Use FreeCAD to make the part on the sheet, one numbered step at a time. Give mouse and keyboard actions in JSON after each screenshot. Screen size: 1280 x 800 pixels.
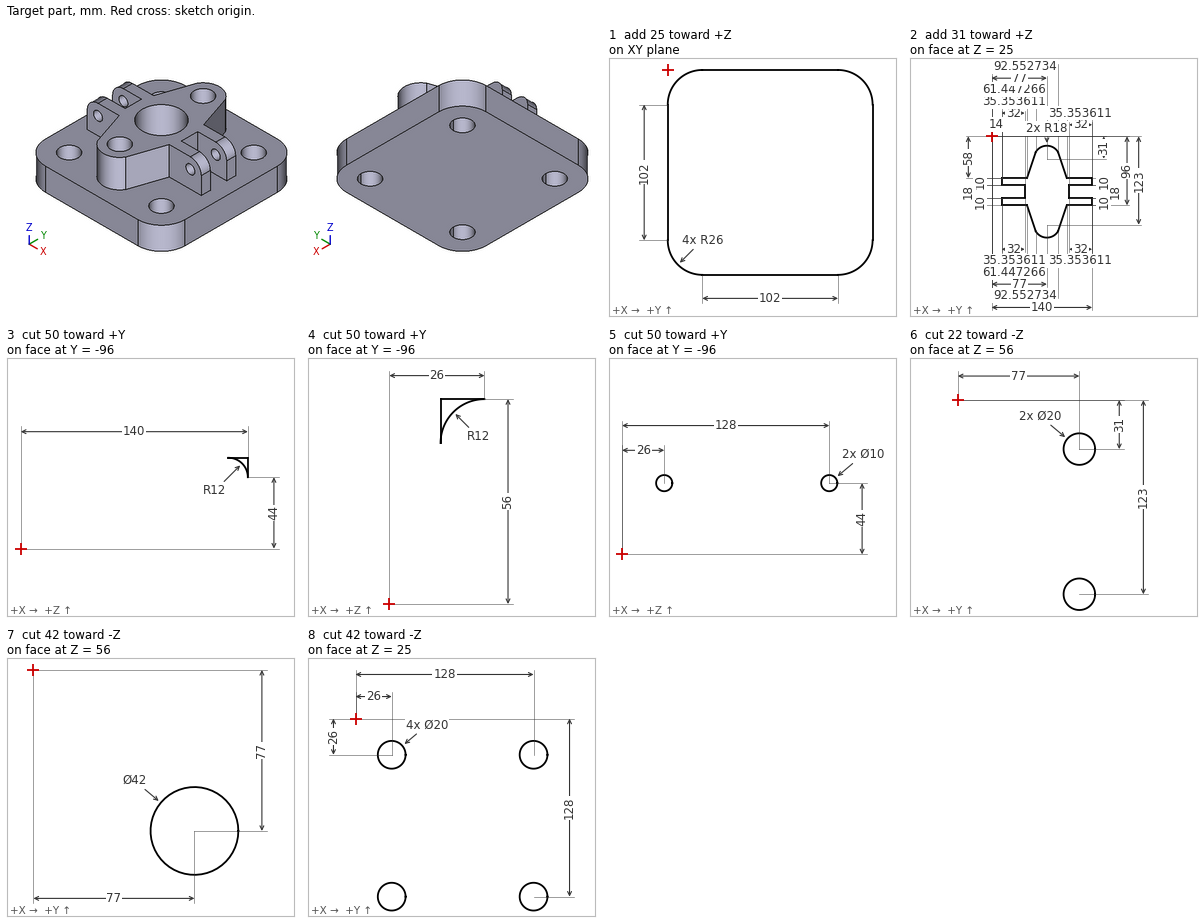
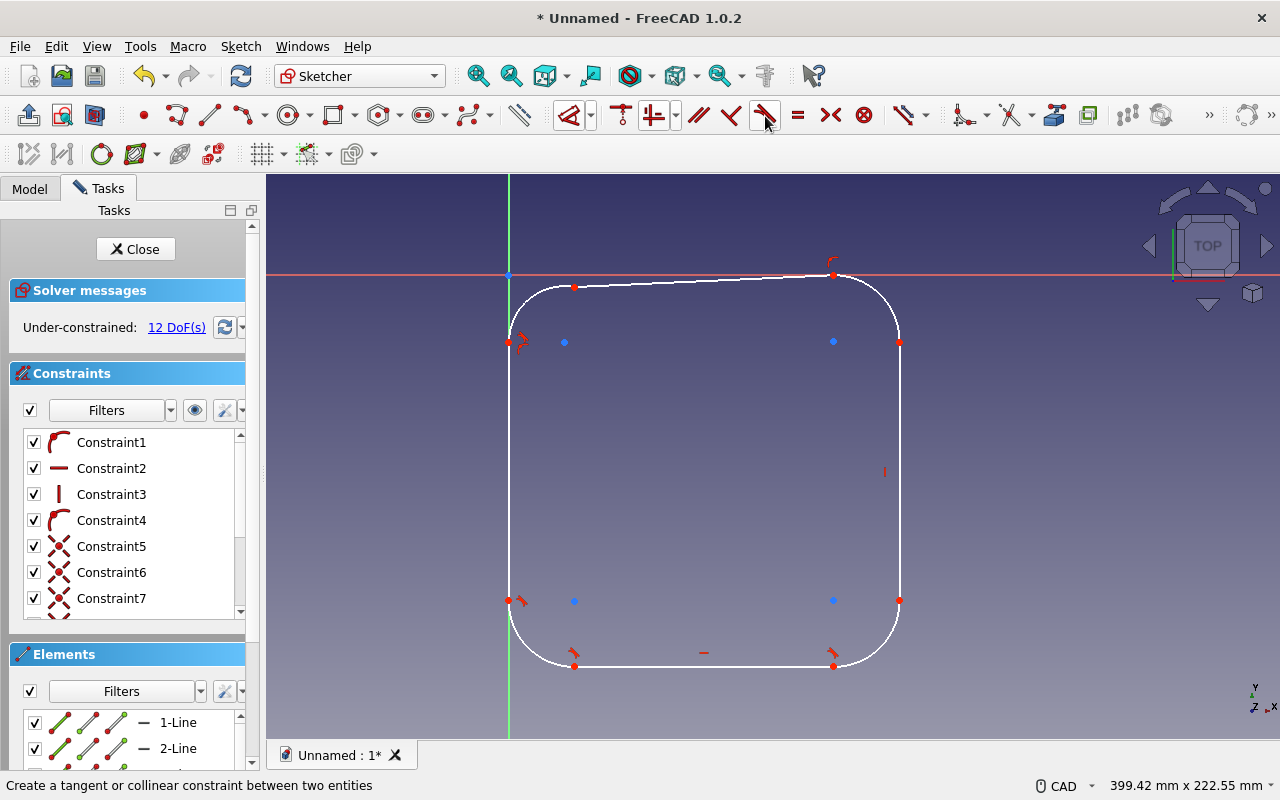
{"action": "left_click", "coordinate": [900, 523]}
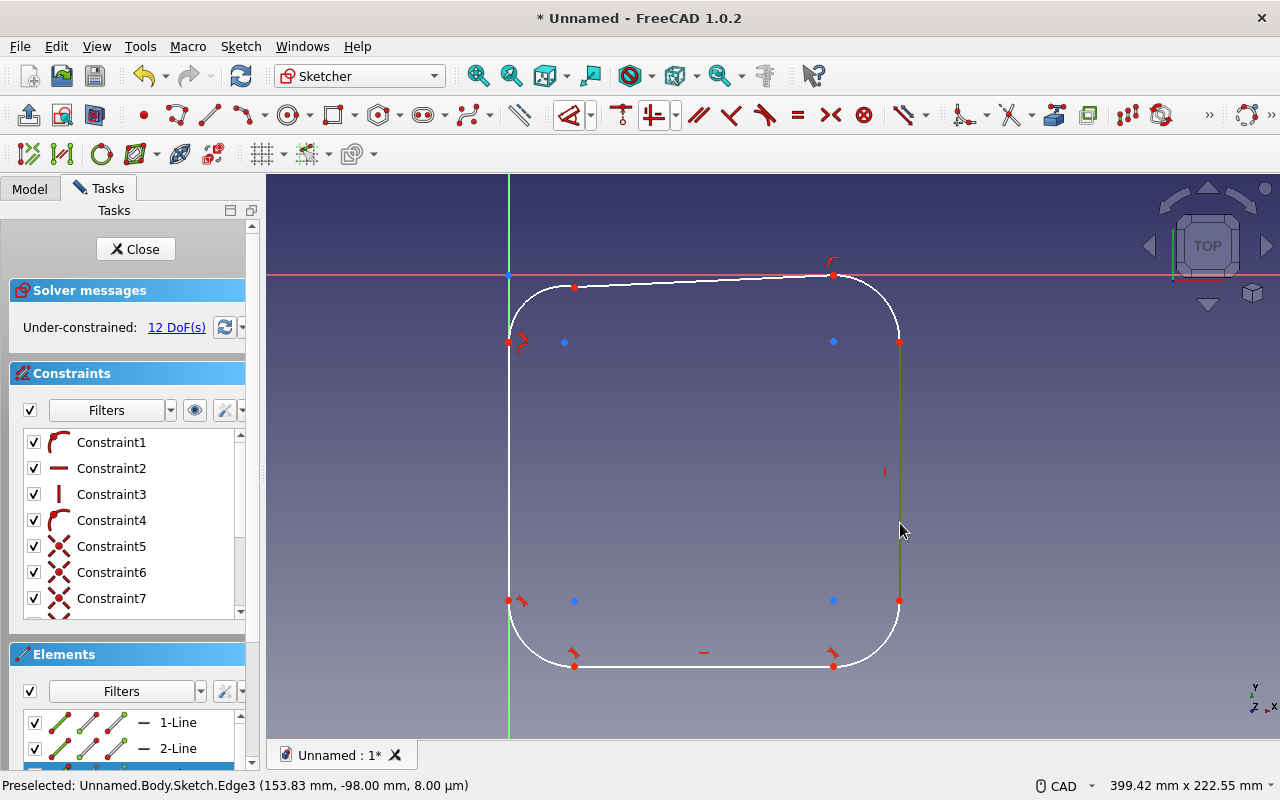
{"action": "left_click", "coordinate": [863, 660]}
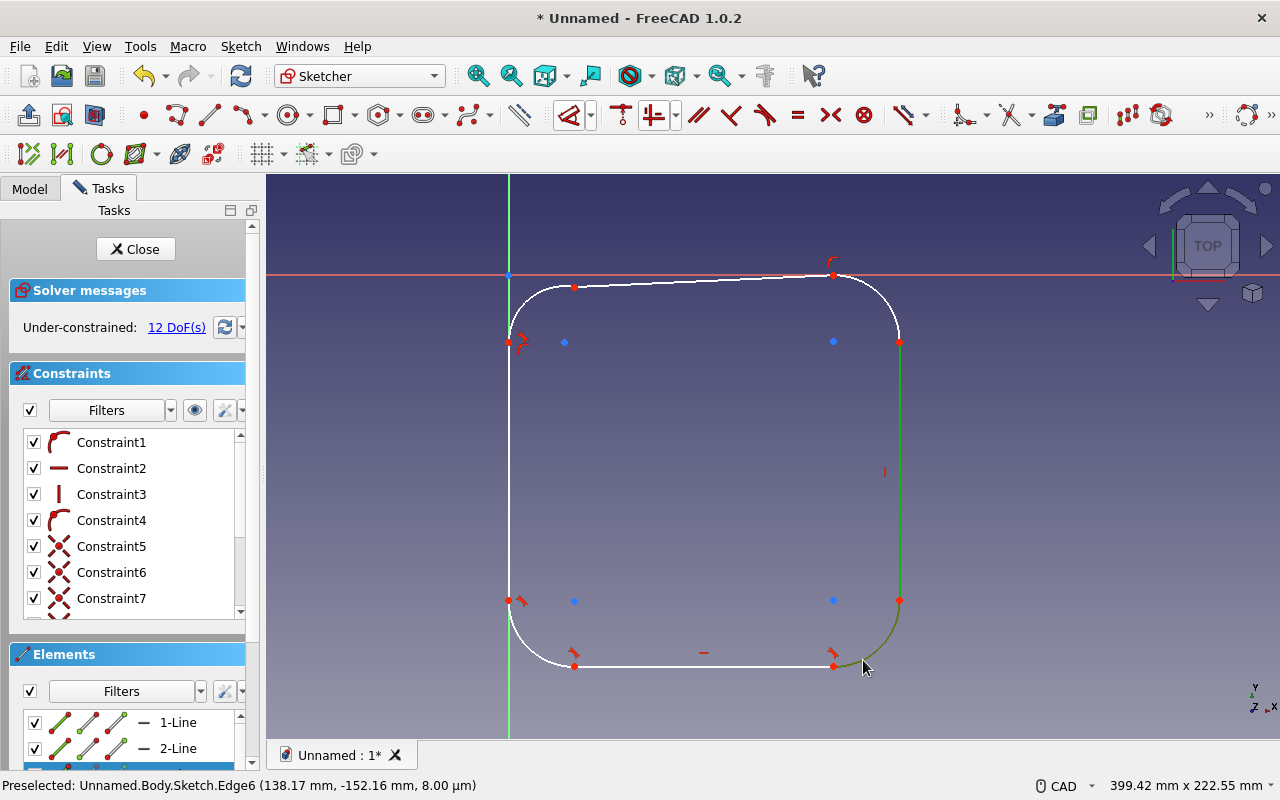
{"action": "left_click", "coordinate": [765, 116]}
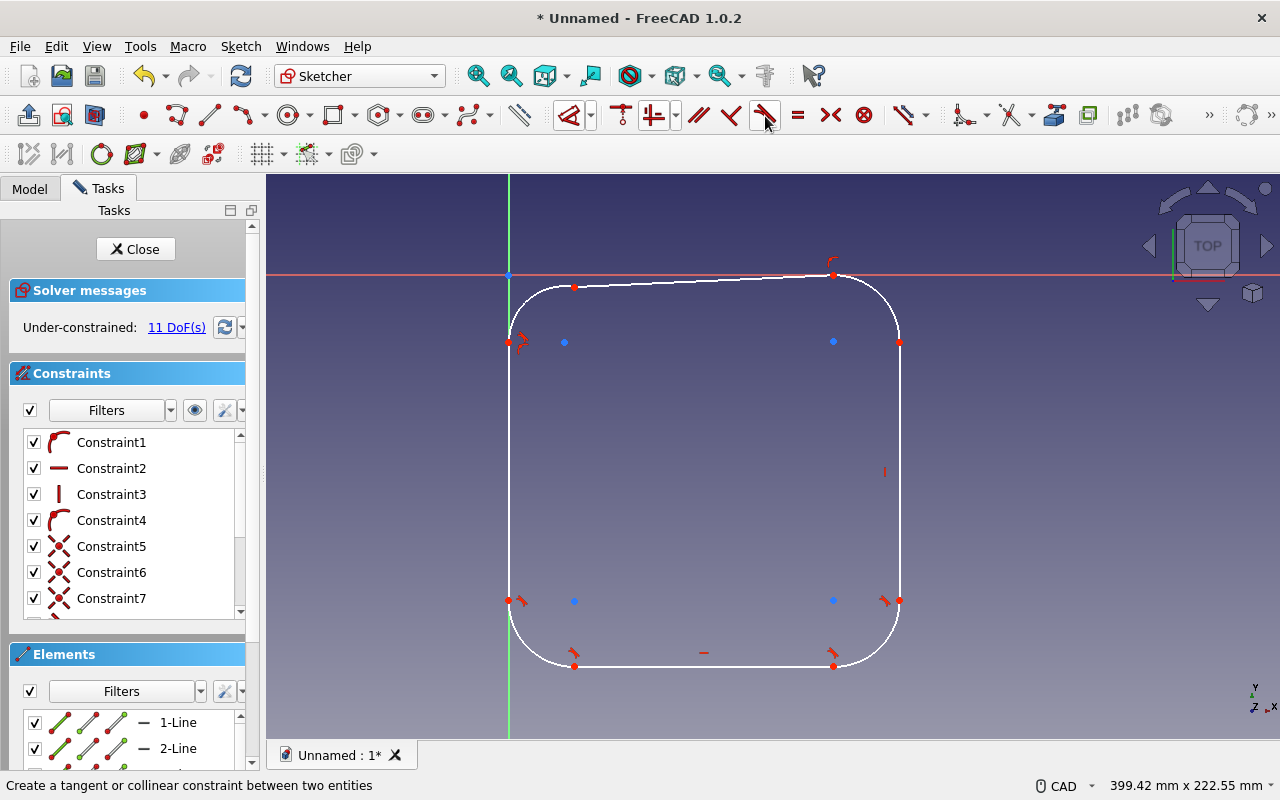
{"action": "left_click", "coordinate": [900, 523]}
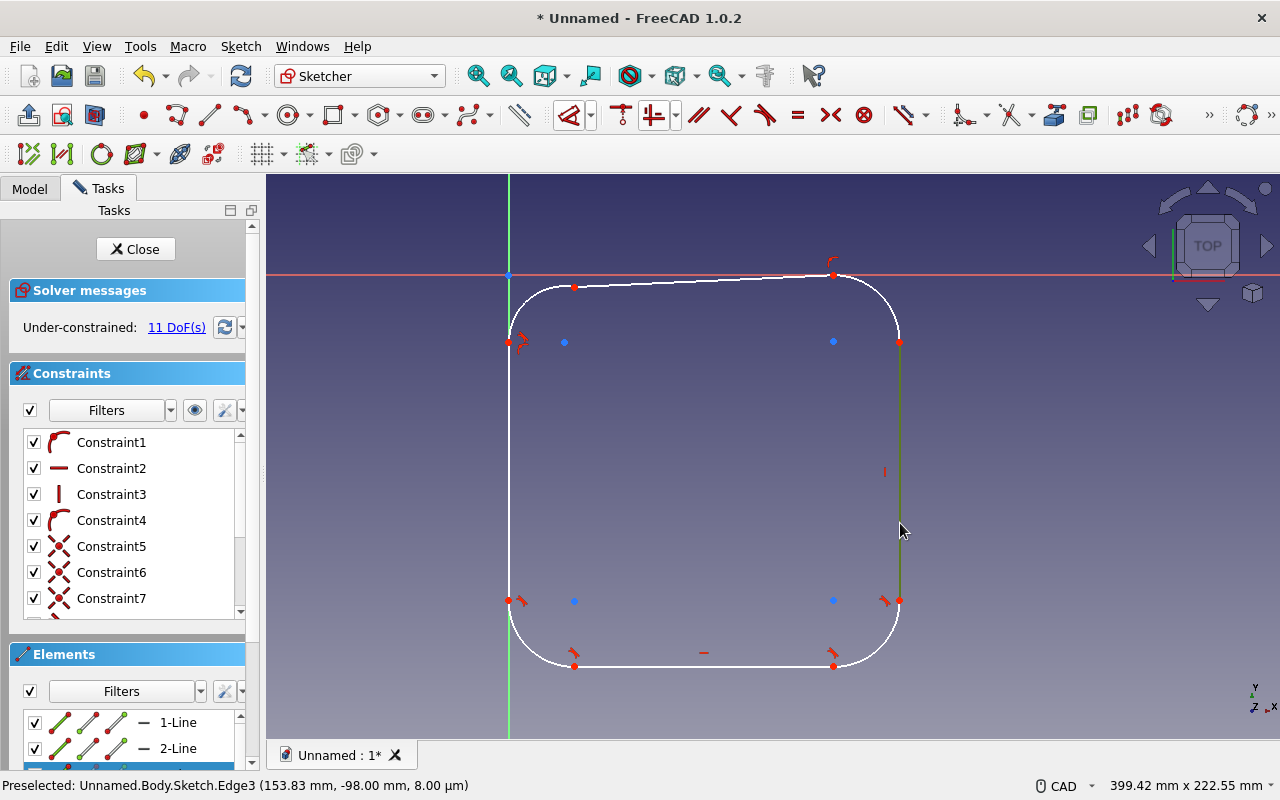
{"action": "left_click", "coordinate": [893, 312]}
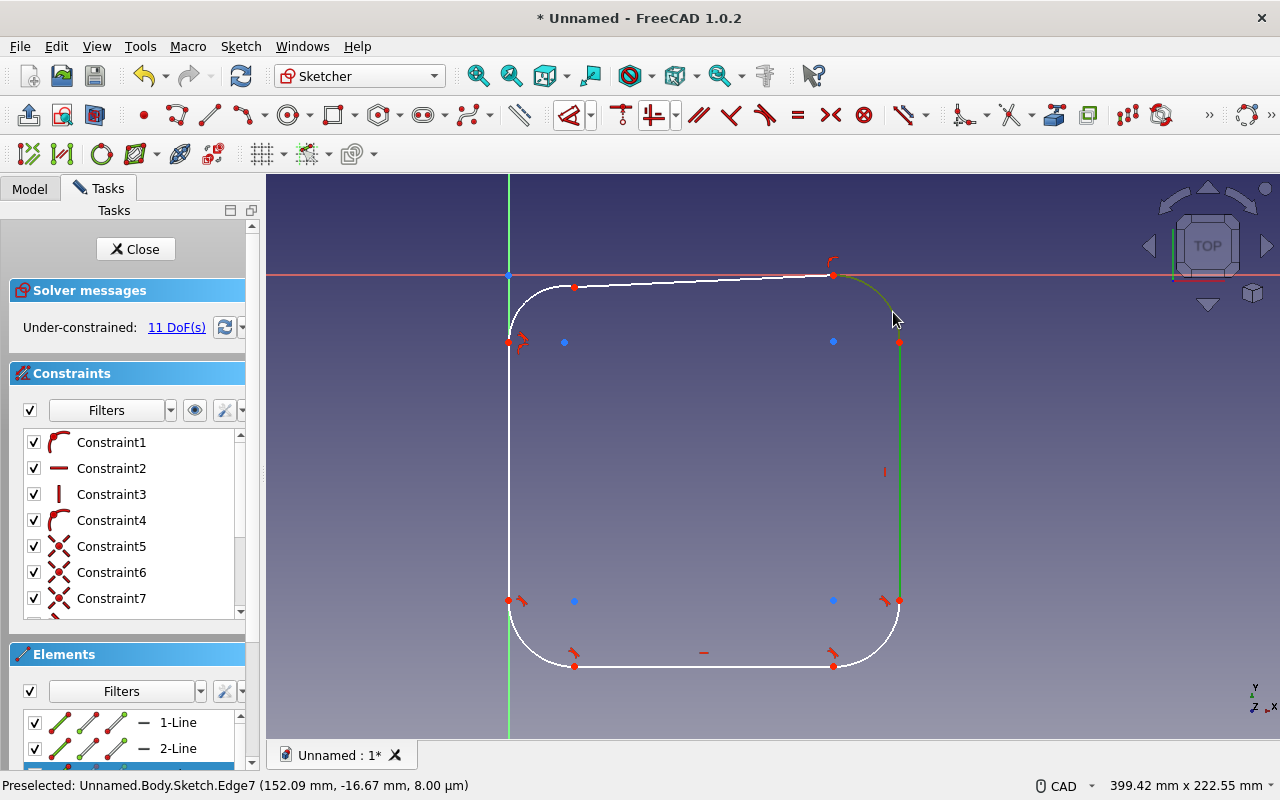
{"action": "left_click", "coordinate": [765, 116]}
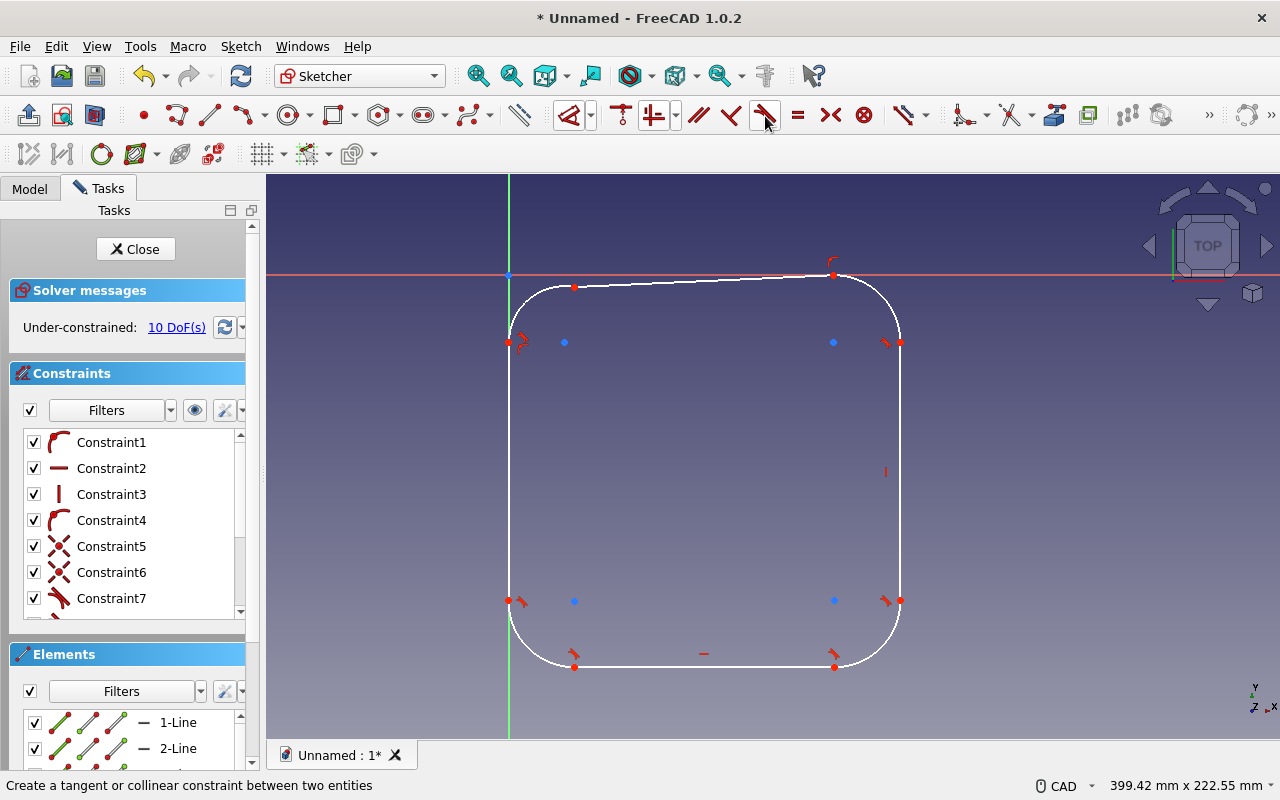
{"action": "left_click", "coordinate": [756, 279]}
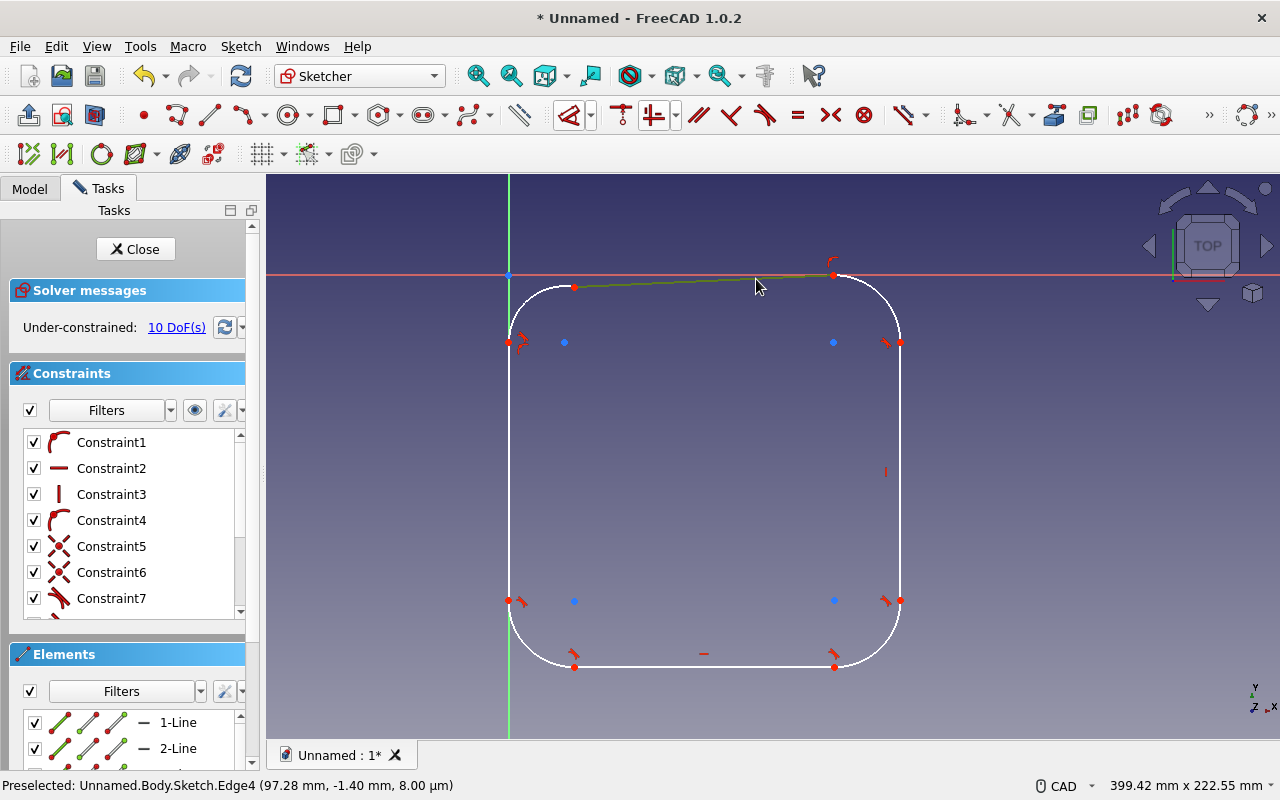
{"action": "left_click", "coordinate": [893, 312]}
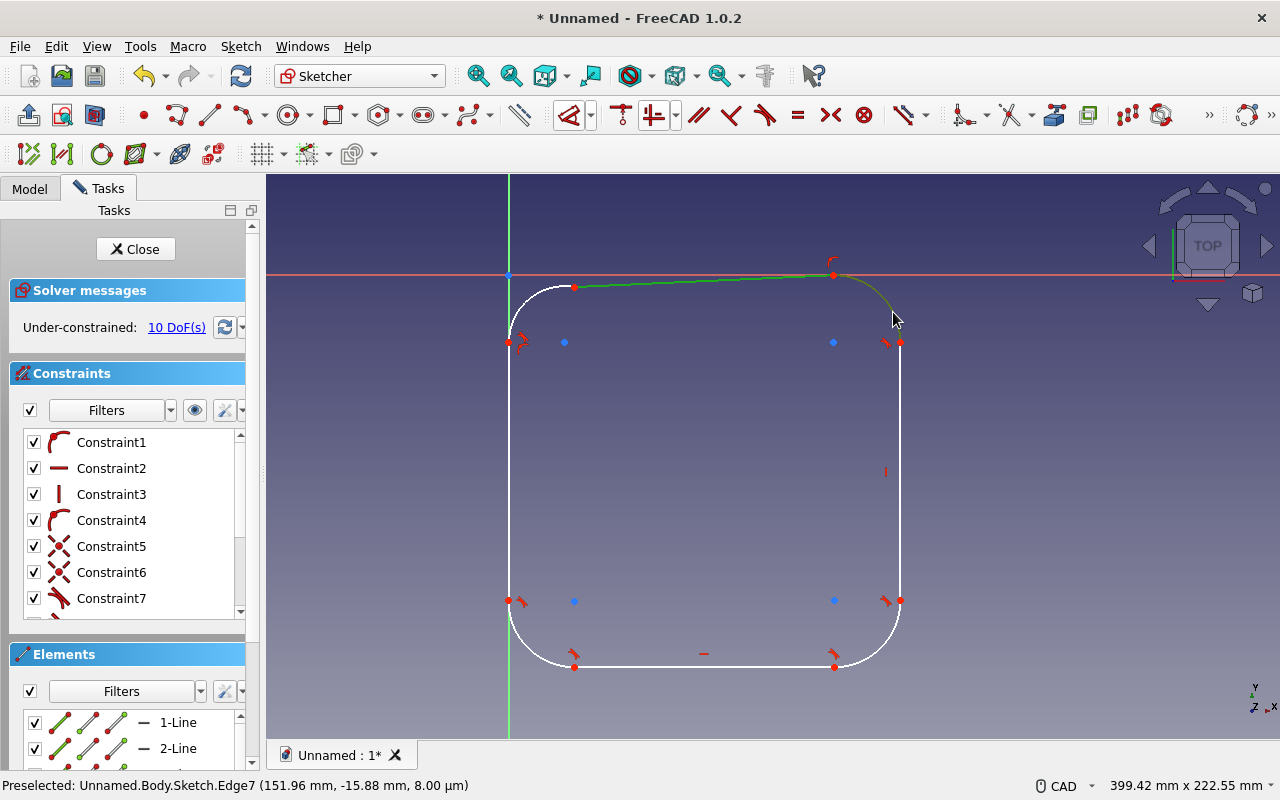
{"action": "left_click", "coordinate": [765, 116]}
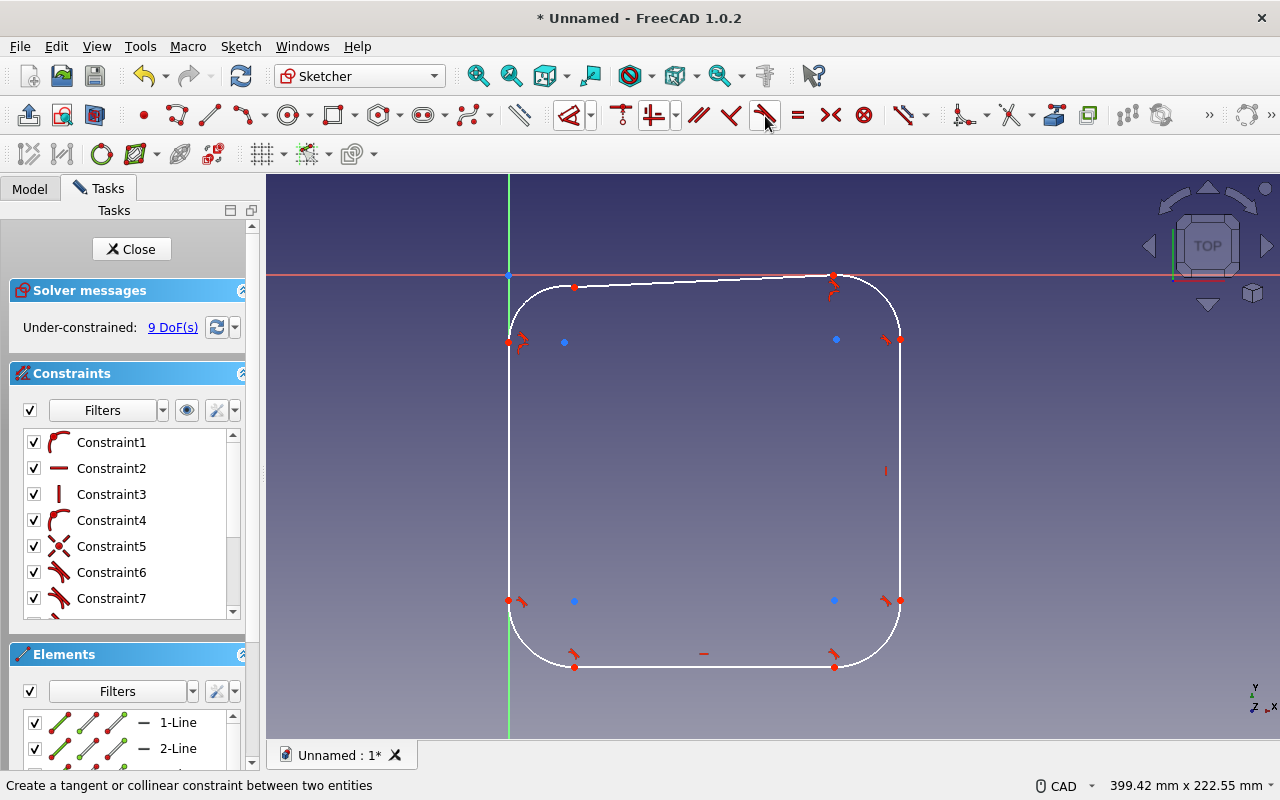
{"action": "left_click", "coordinate": [756, 279]}